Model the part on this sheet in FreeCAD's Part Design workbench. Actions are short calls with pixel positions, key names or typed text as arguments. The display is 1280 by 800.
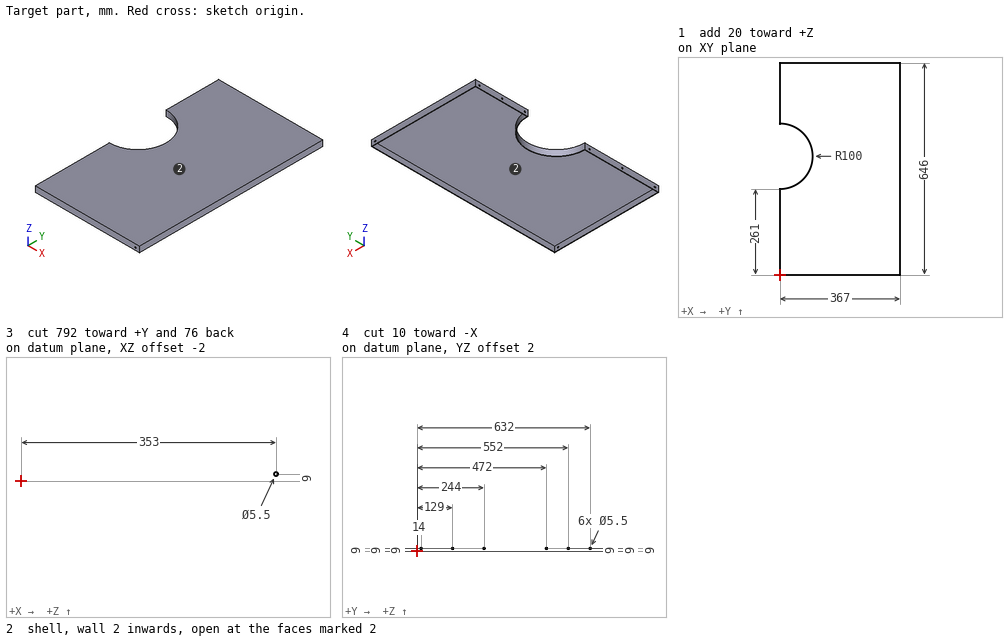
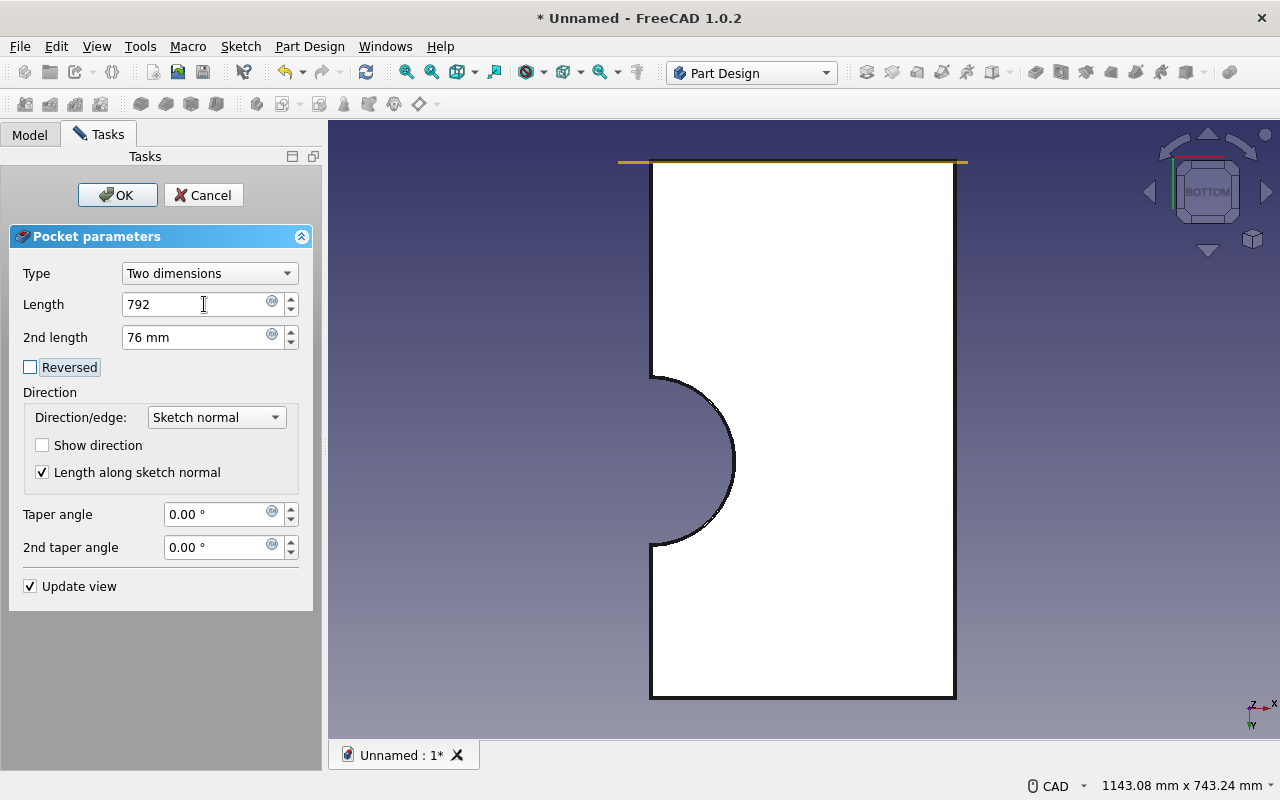
click(118, 195)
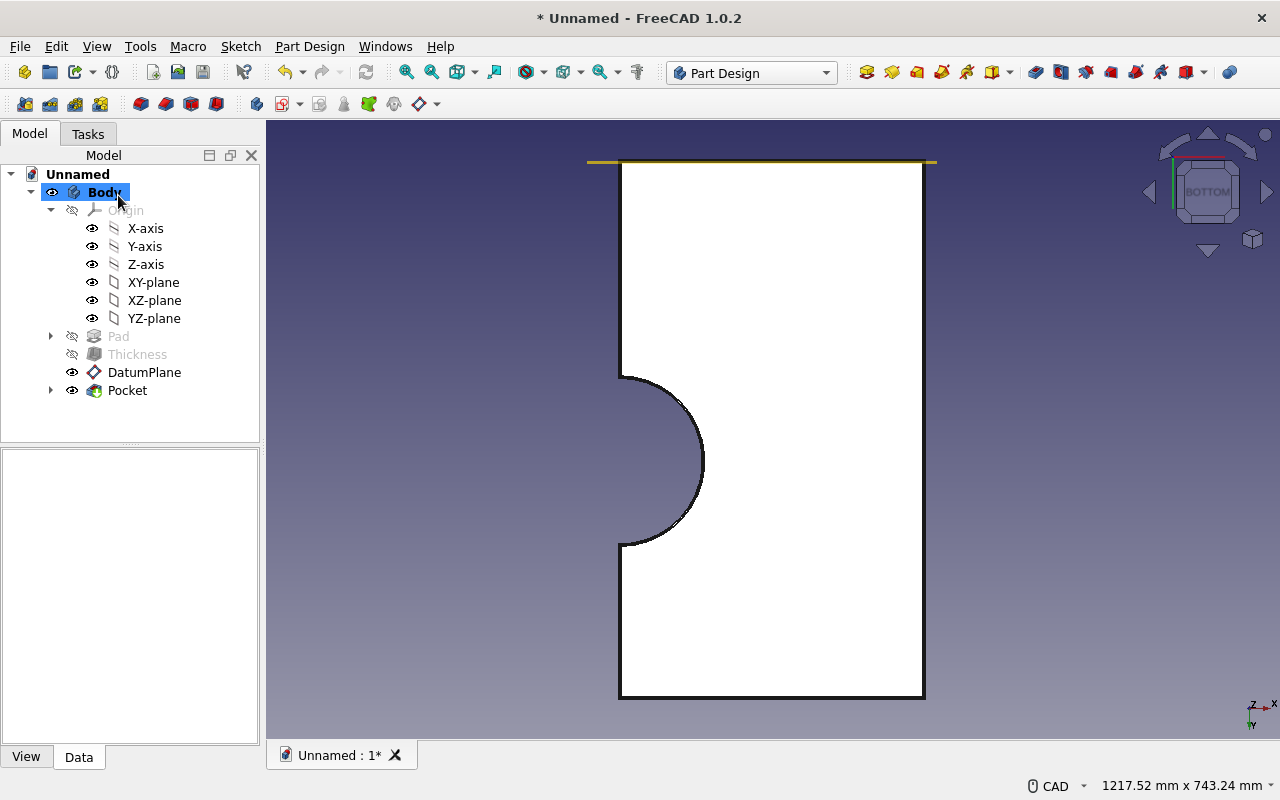
click(117, 372)
key(space)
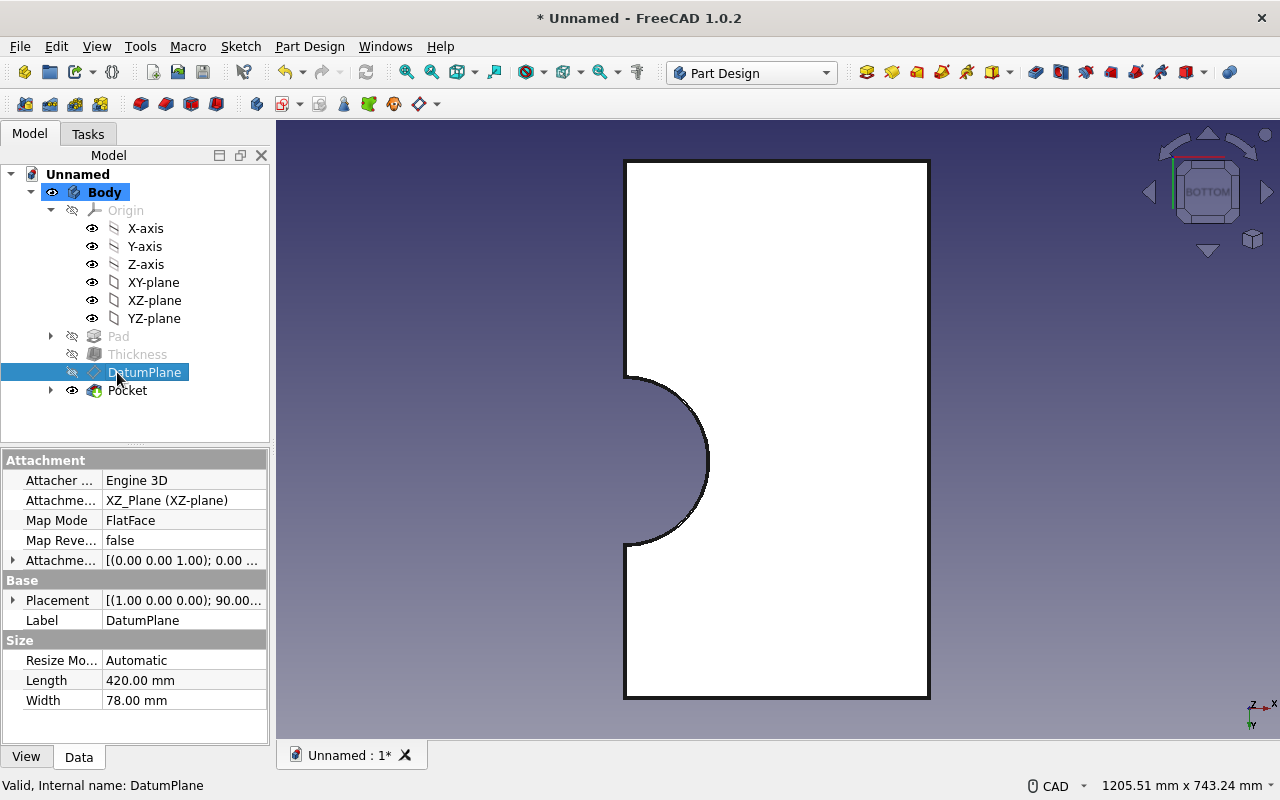
click(137, 318)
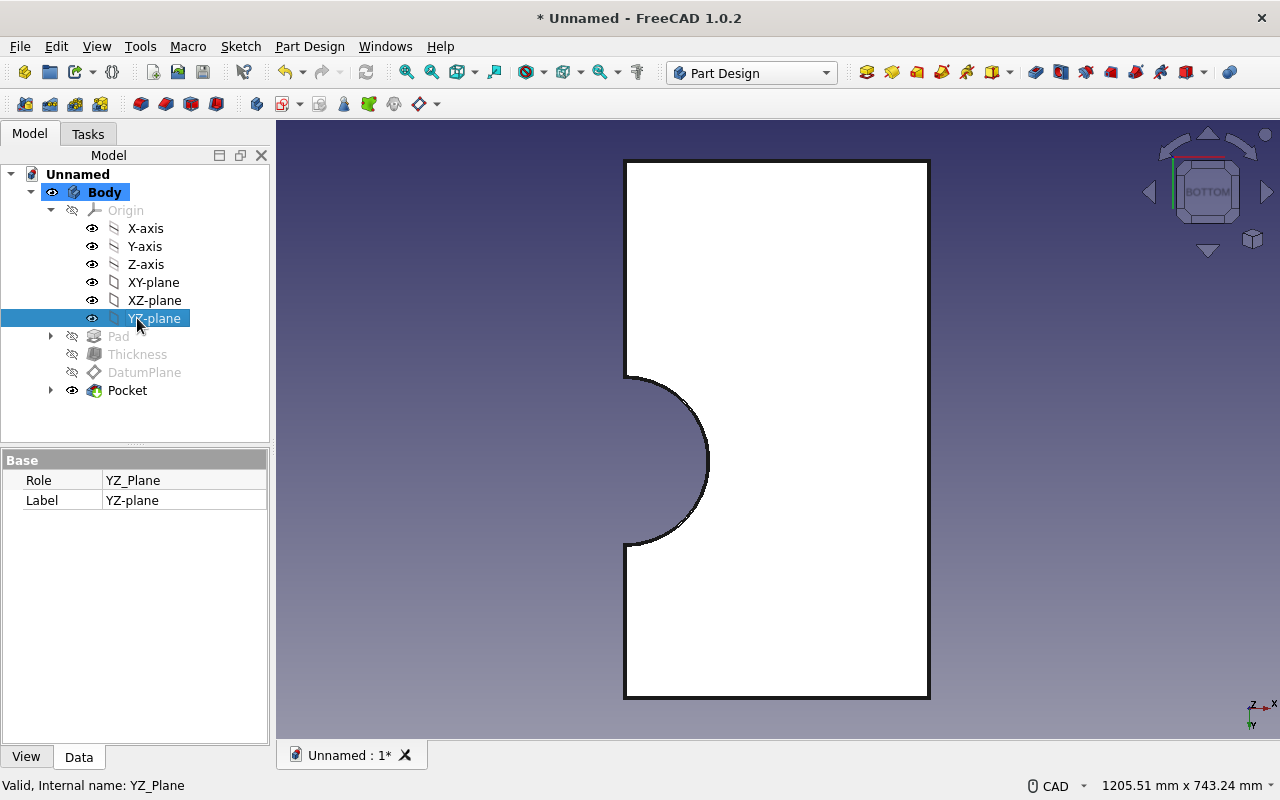
click(418, 104)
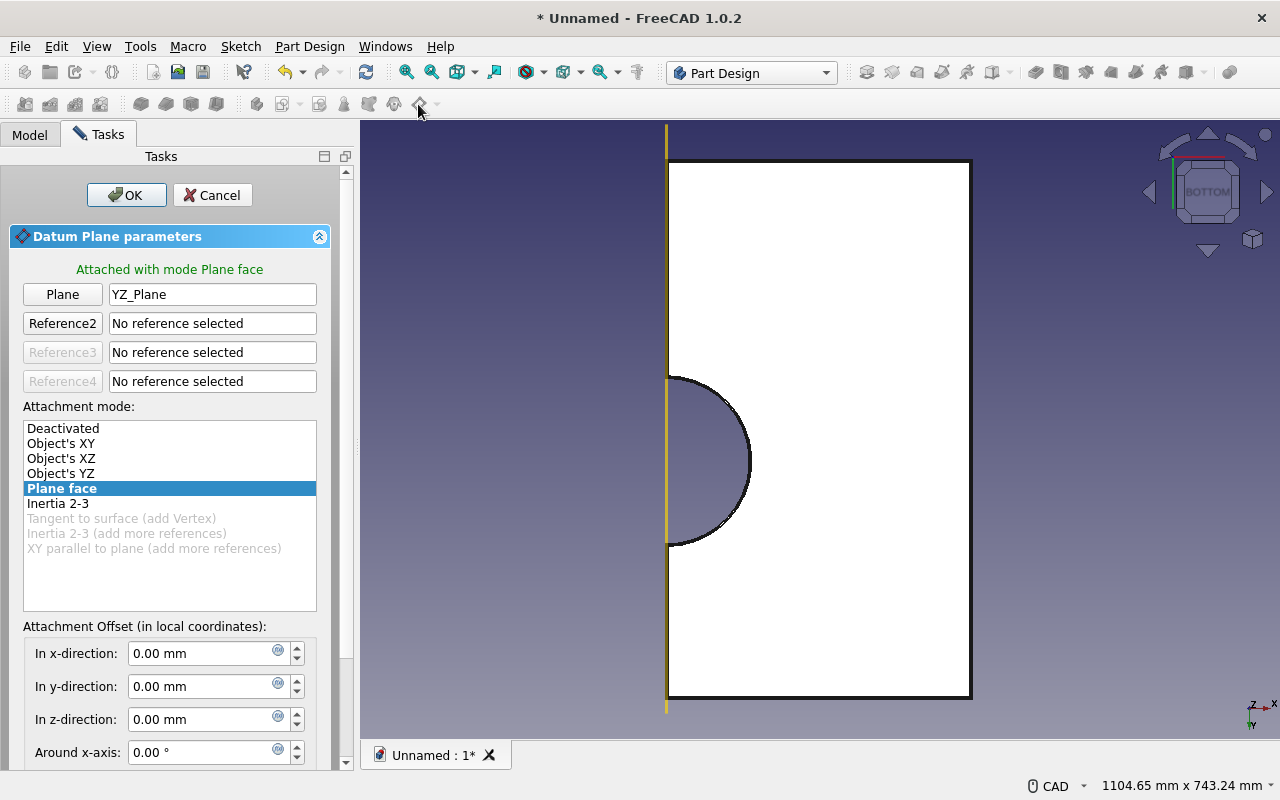
triple_click(210, 720)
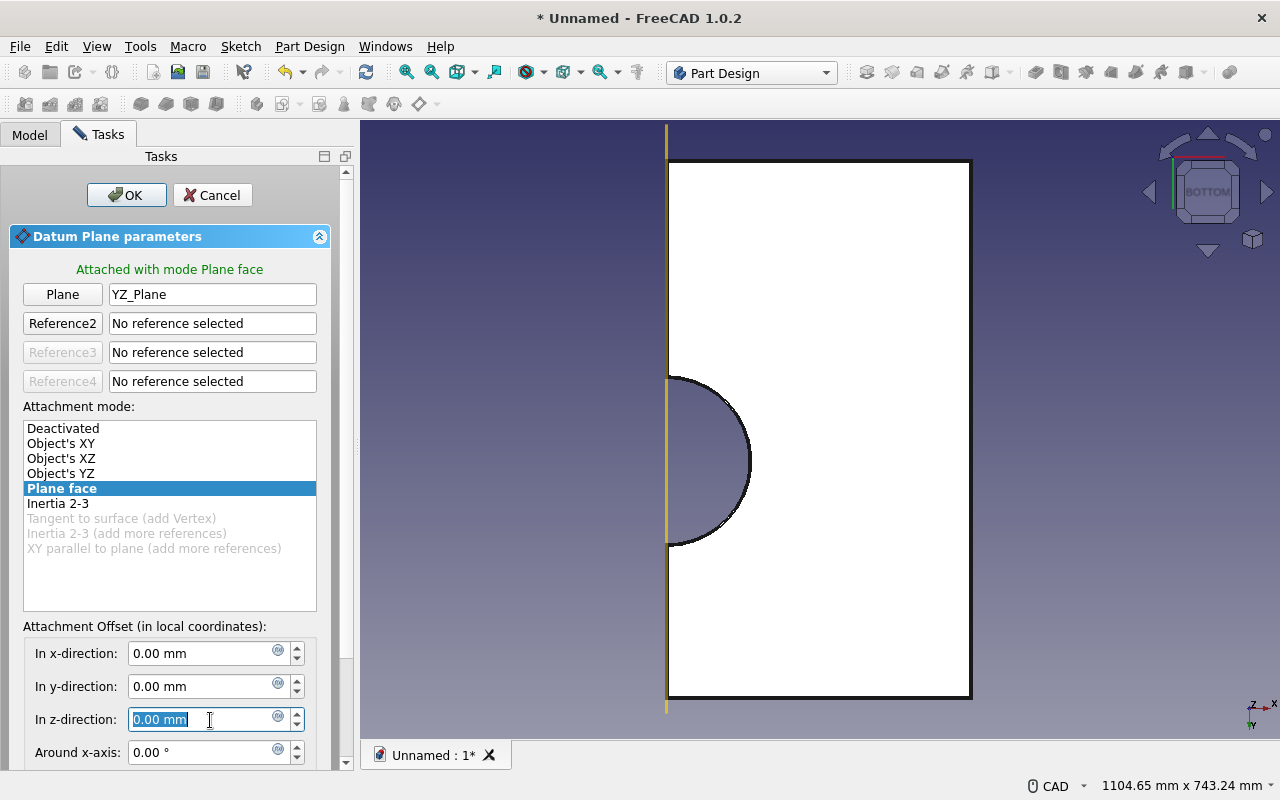
text(2)
key(Tab)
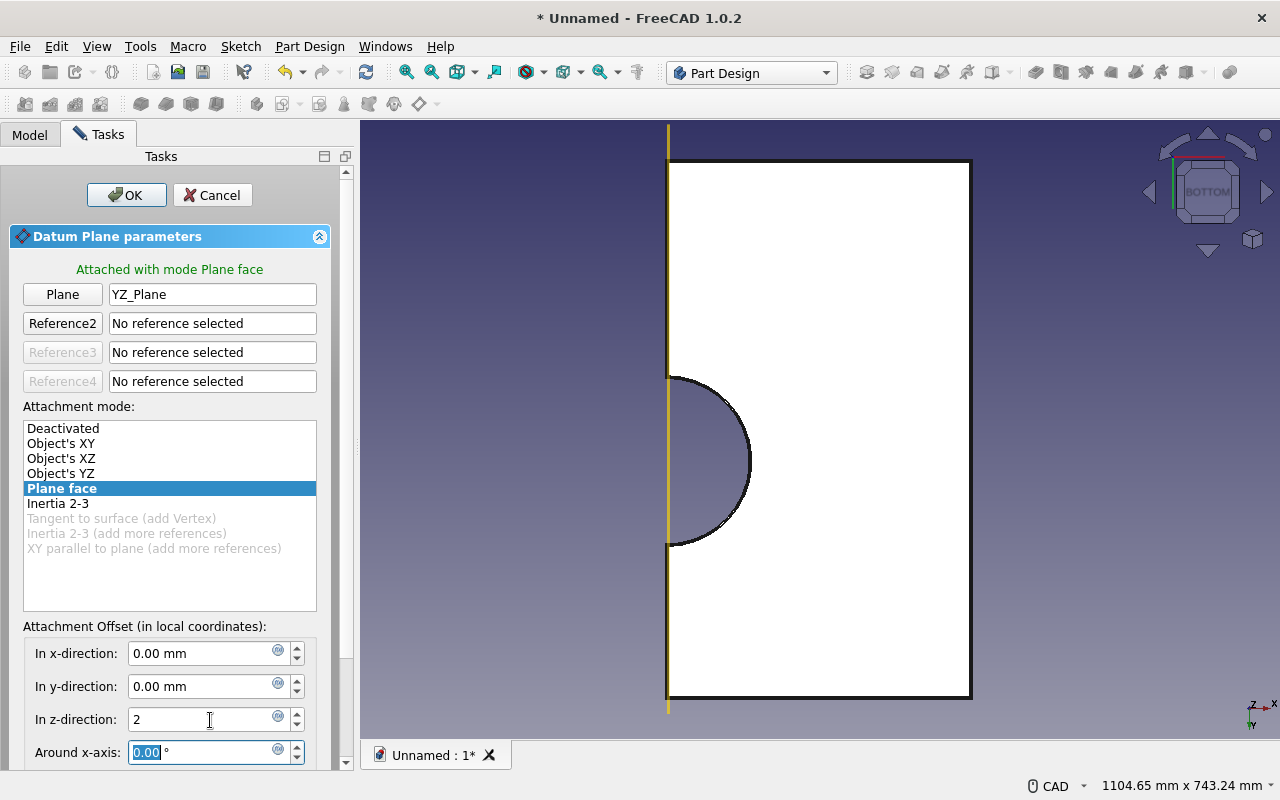
click(127, 195)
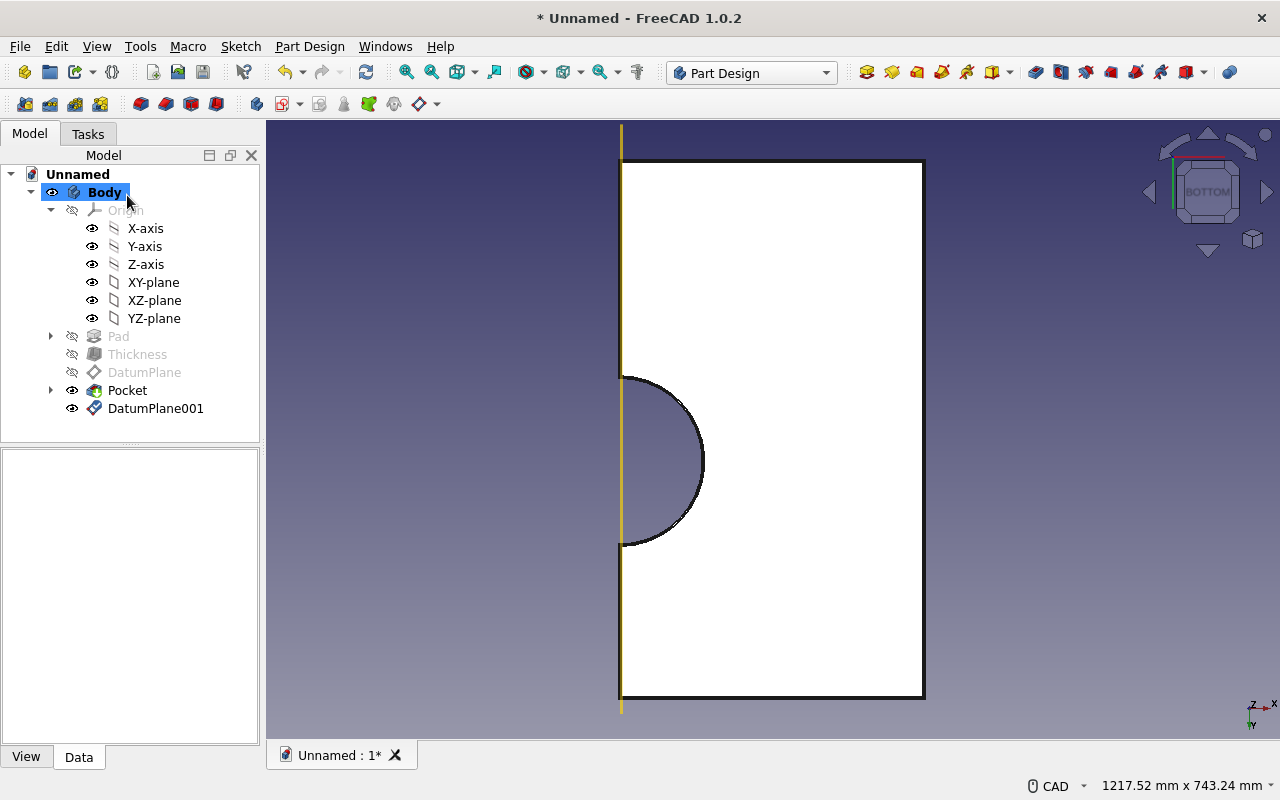
click(117, 408)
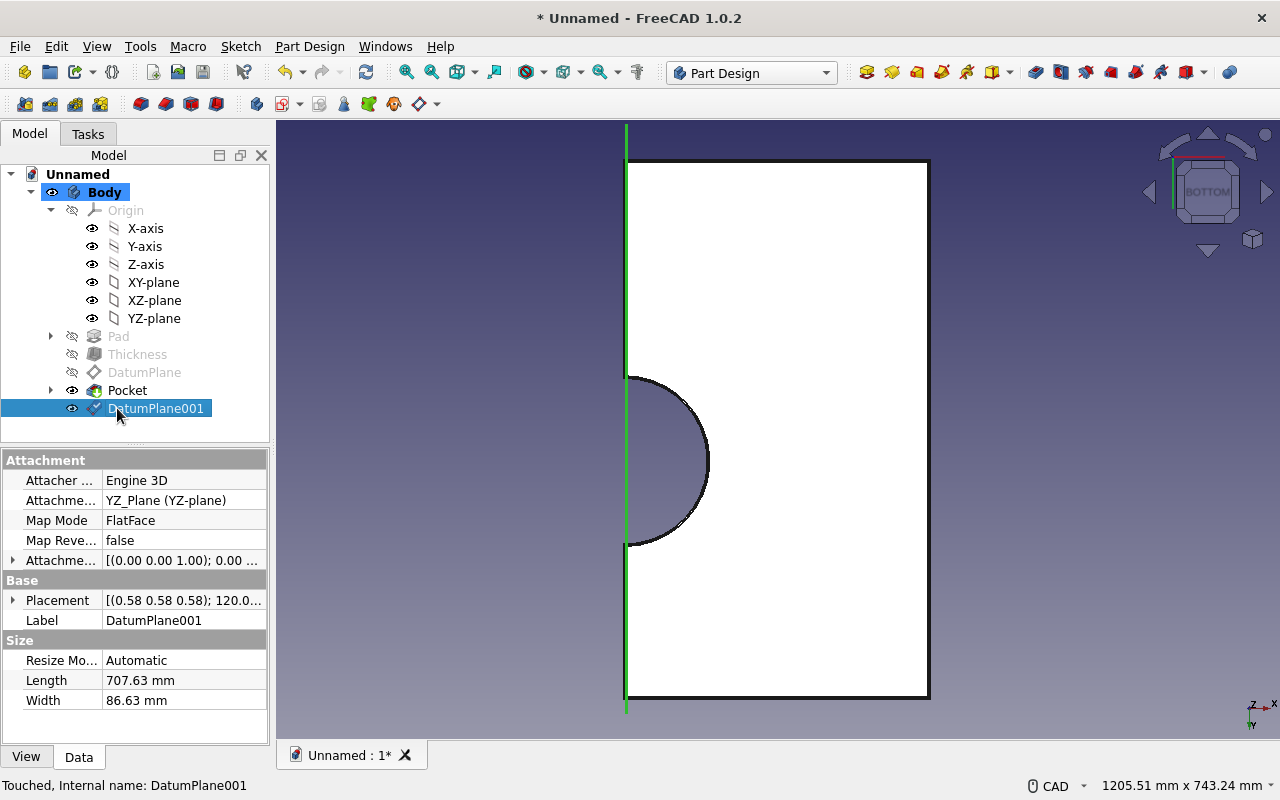
click(282, 104)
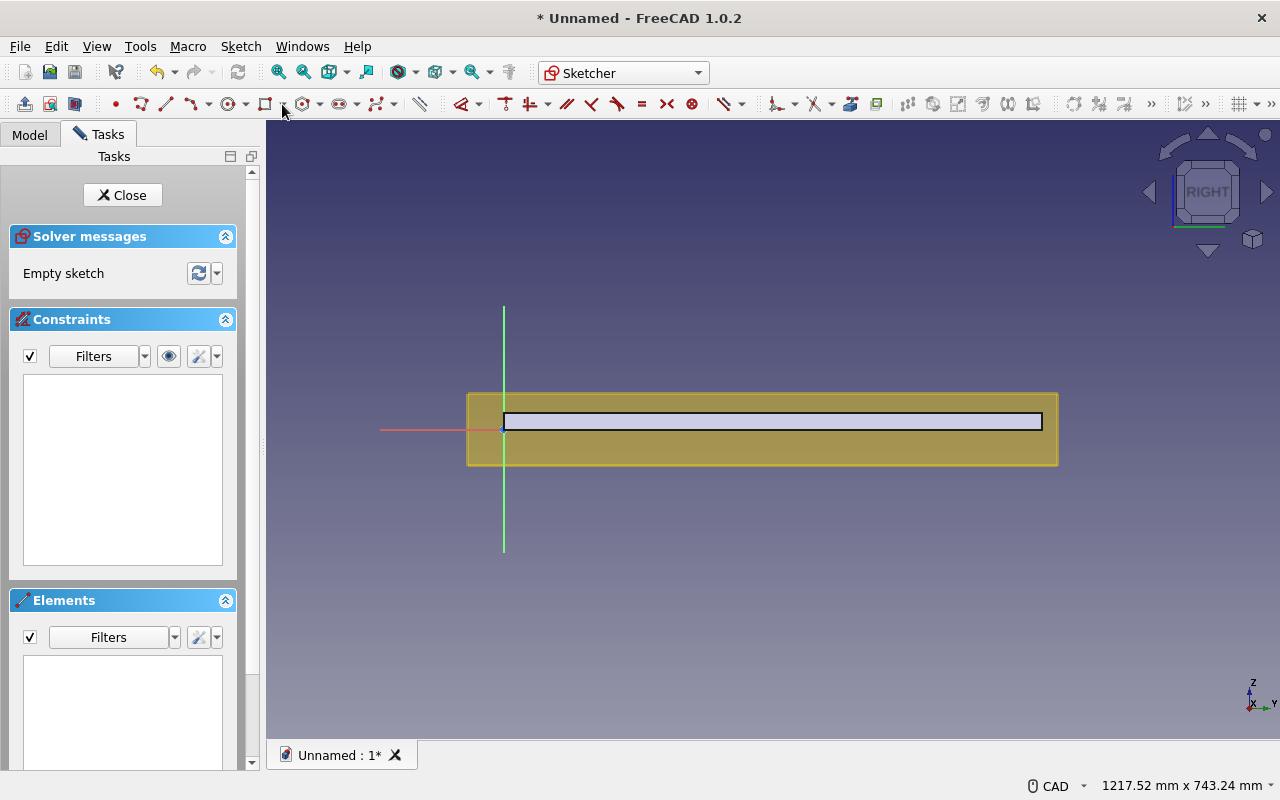
click(75, 104)